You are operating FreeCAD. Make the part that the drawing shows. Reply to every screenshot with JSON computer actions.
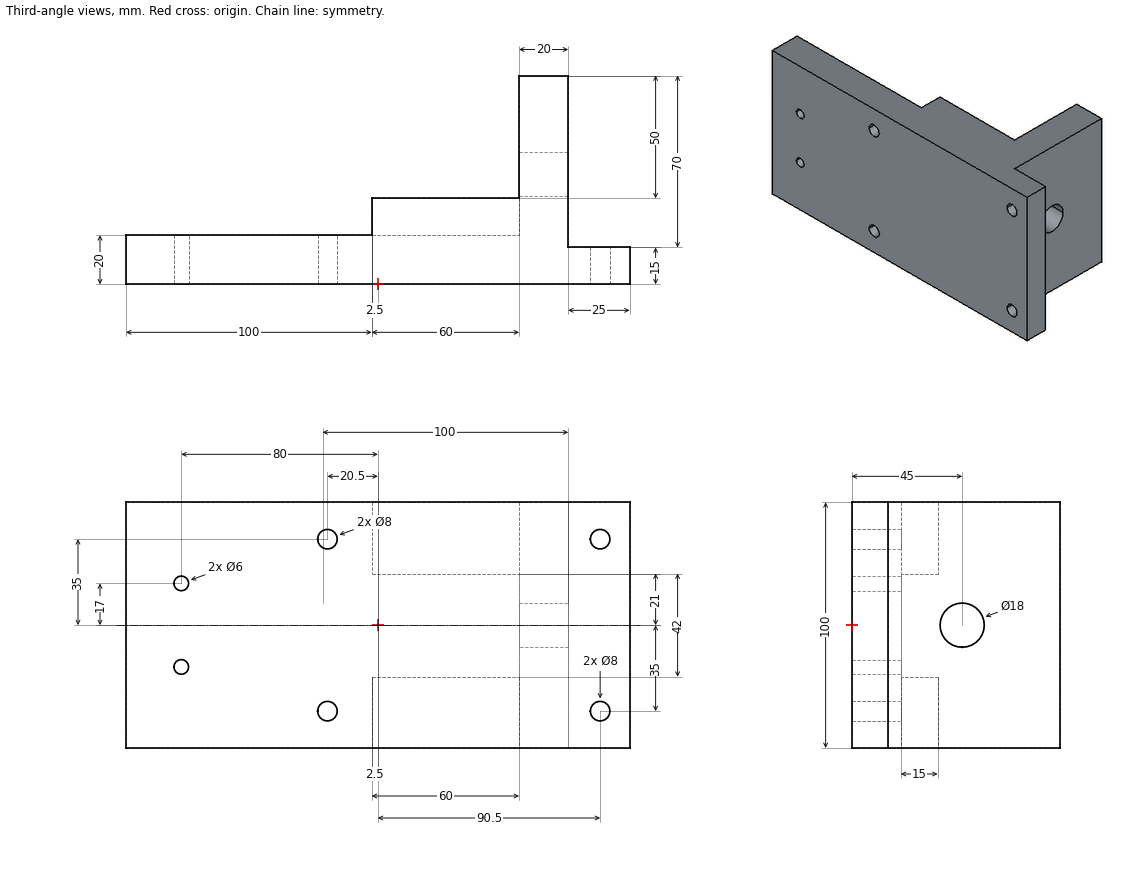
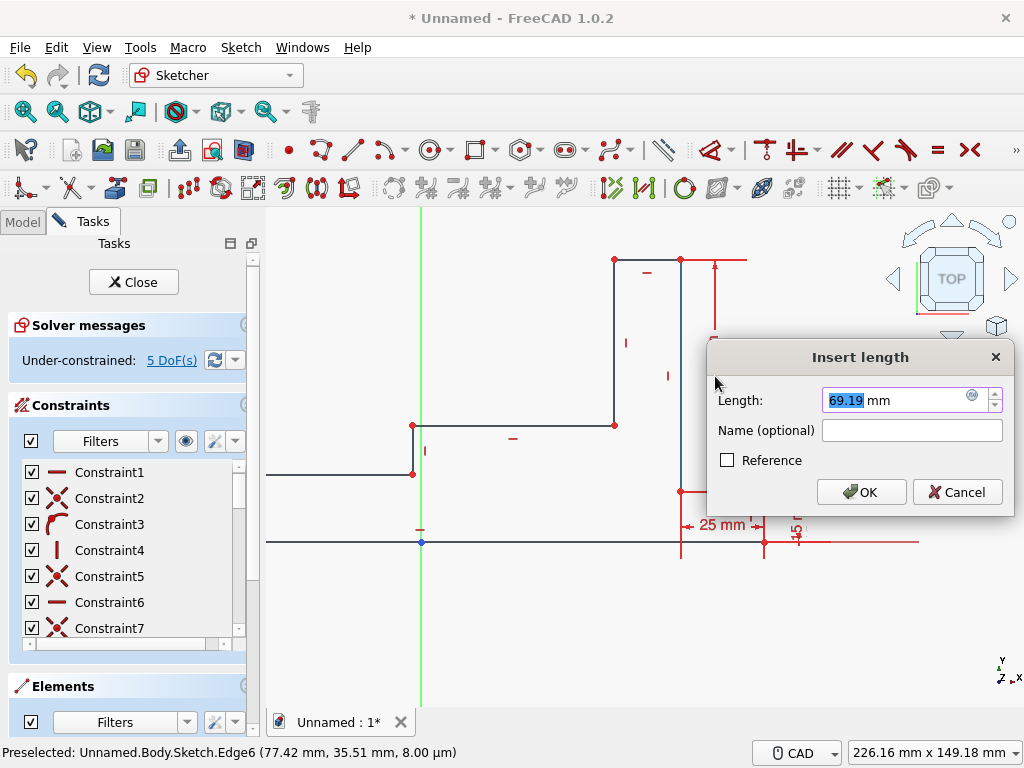
{"action": "type", "text": "70"}
{"action": "key", "text": "Return"}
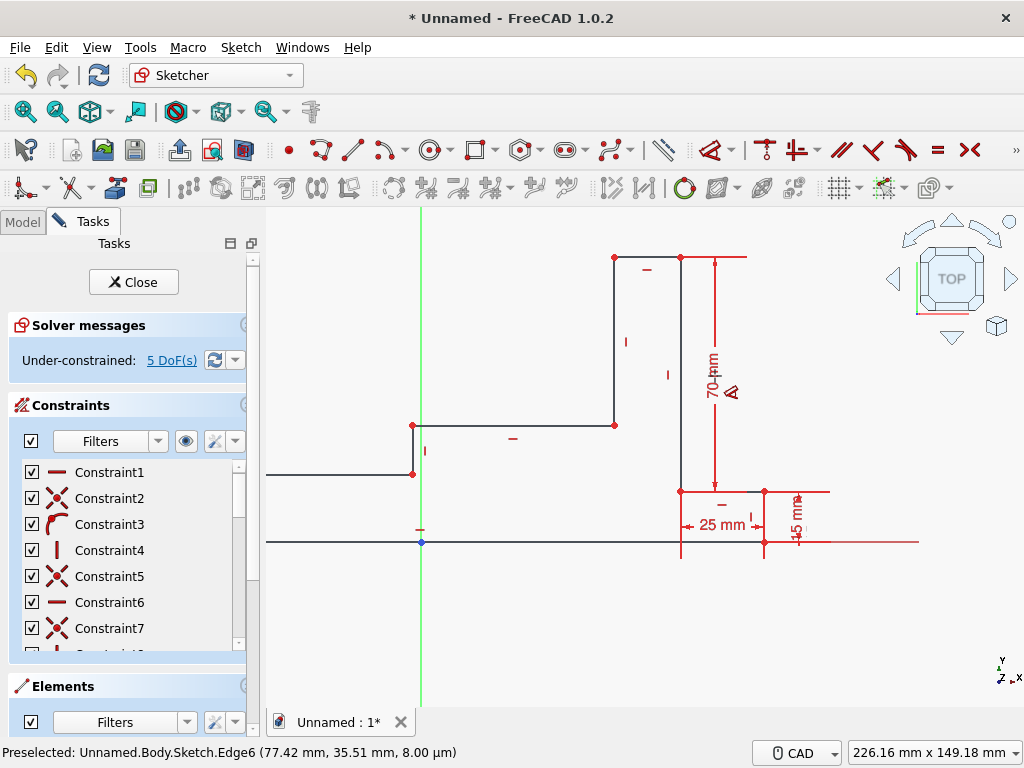
{"action": "left_click", "coordinate": [661, 257]}
{"action": "left_click", "coordinate": [648, 291]}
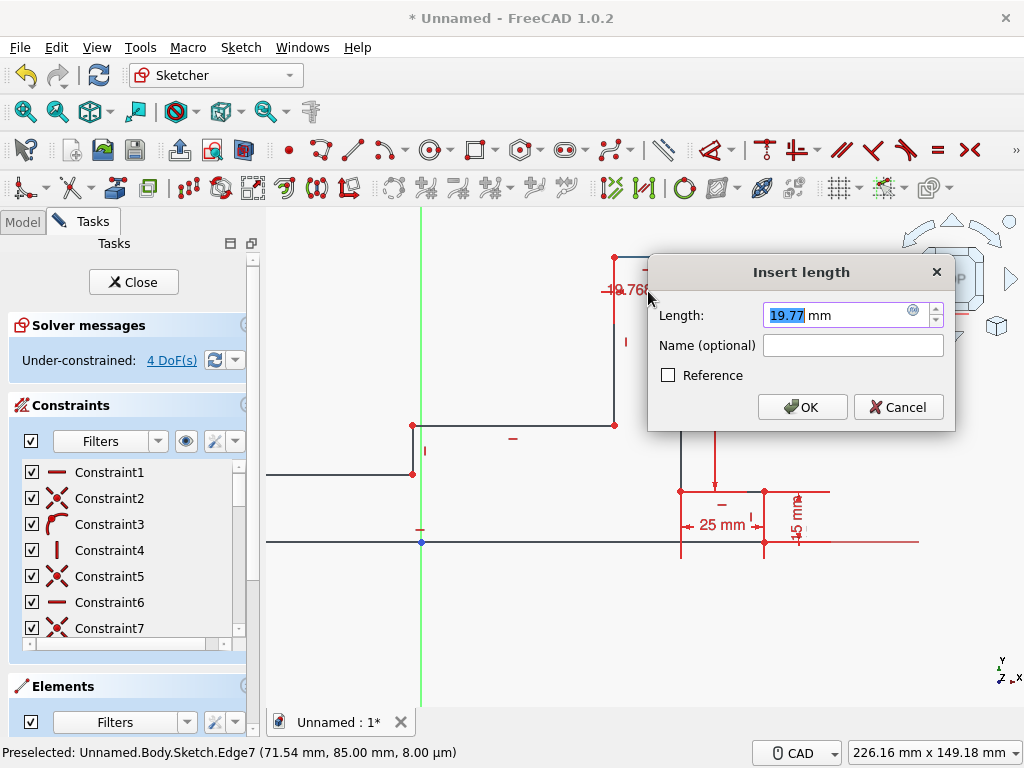
{"action": "type", "text": "20"}
{"action": "key", "text": "Return"}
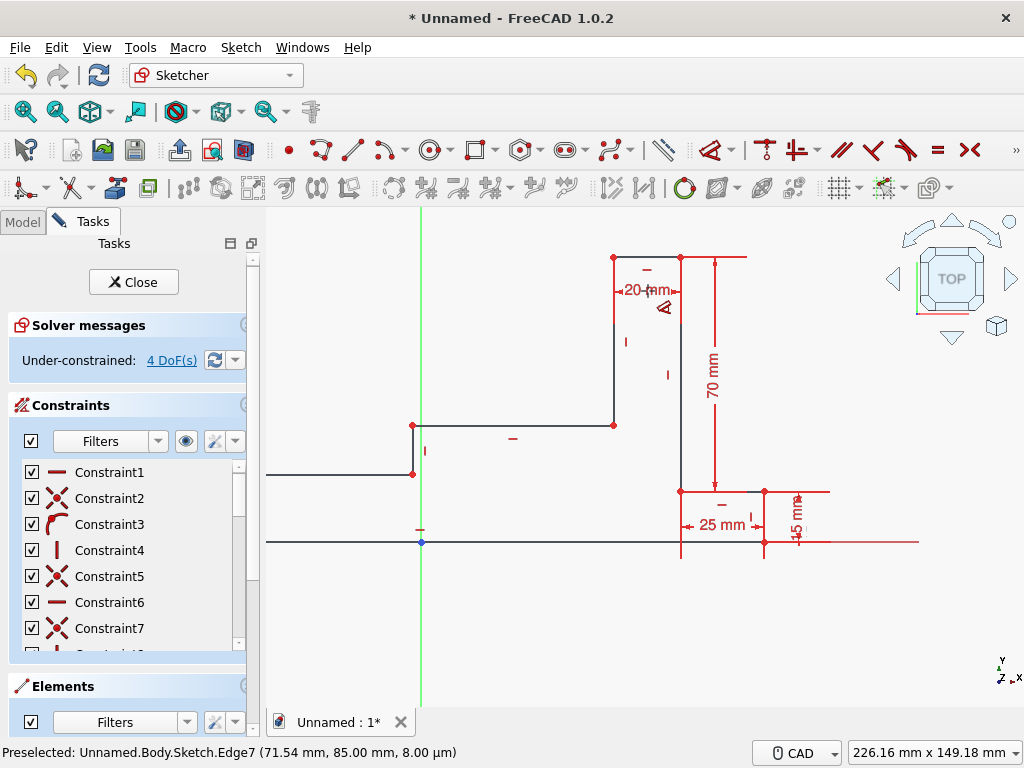
{"action": "left_click", "coordinate": [614, 308]}
{"action": "left_click", "coordinate": [648, 341]}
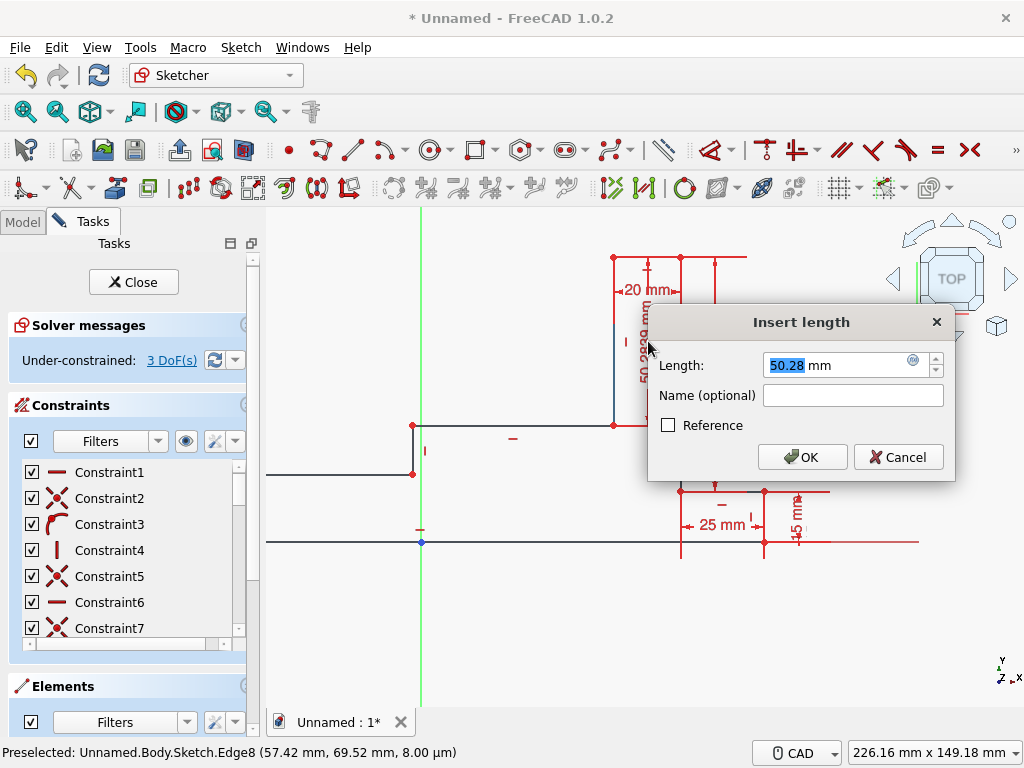
{"action": "type", "text": "50"}
{"action": "key", "text": "Return"}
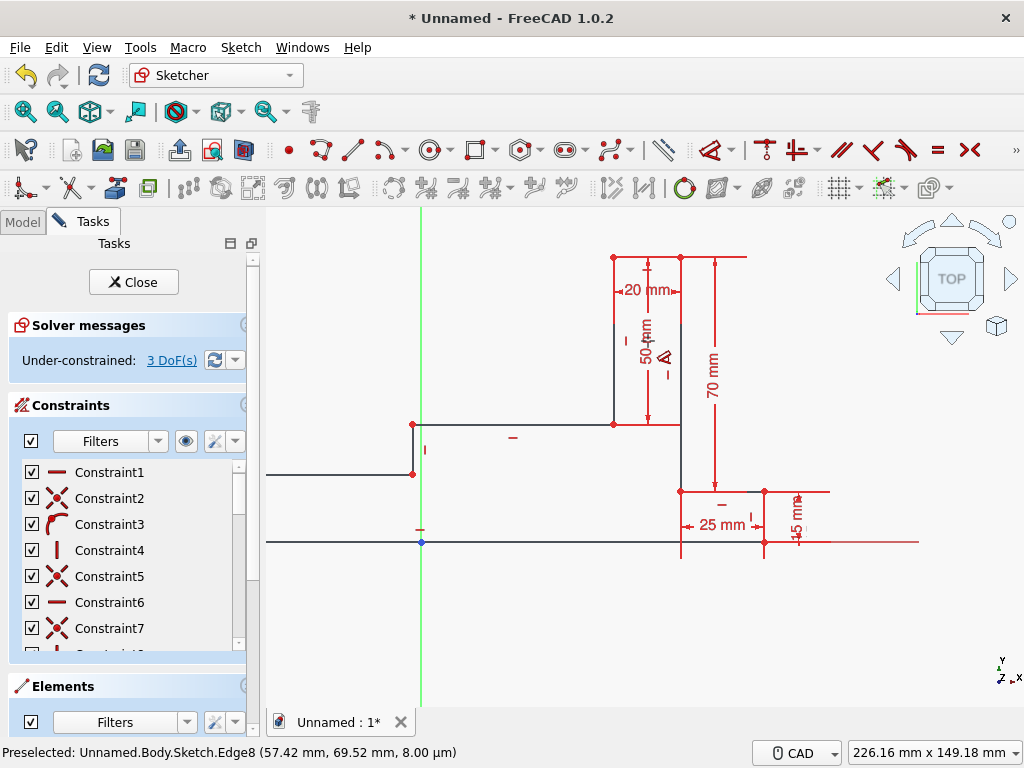
{"action": "left_click", "coordinate": [553, 425]}
{"action": "left_click", "coordinate": [513, 459]}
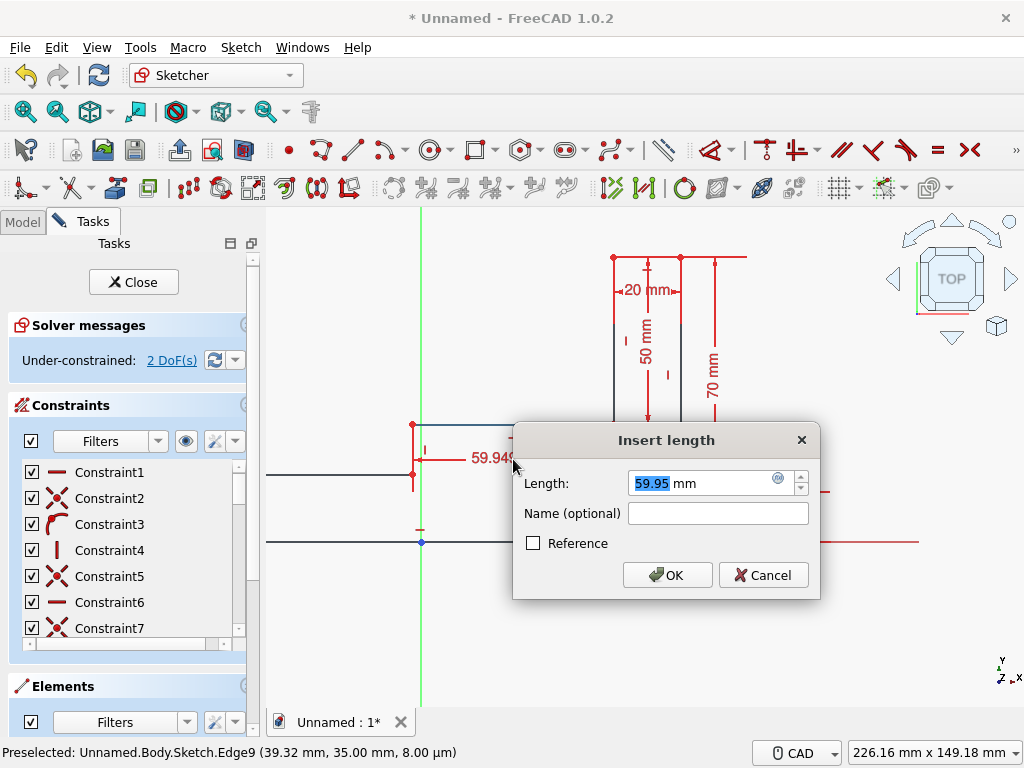
{"action": "type", "text": "60"}
{"action": "key", "text": "Return"}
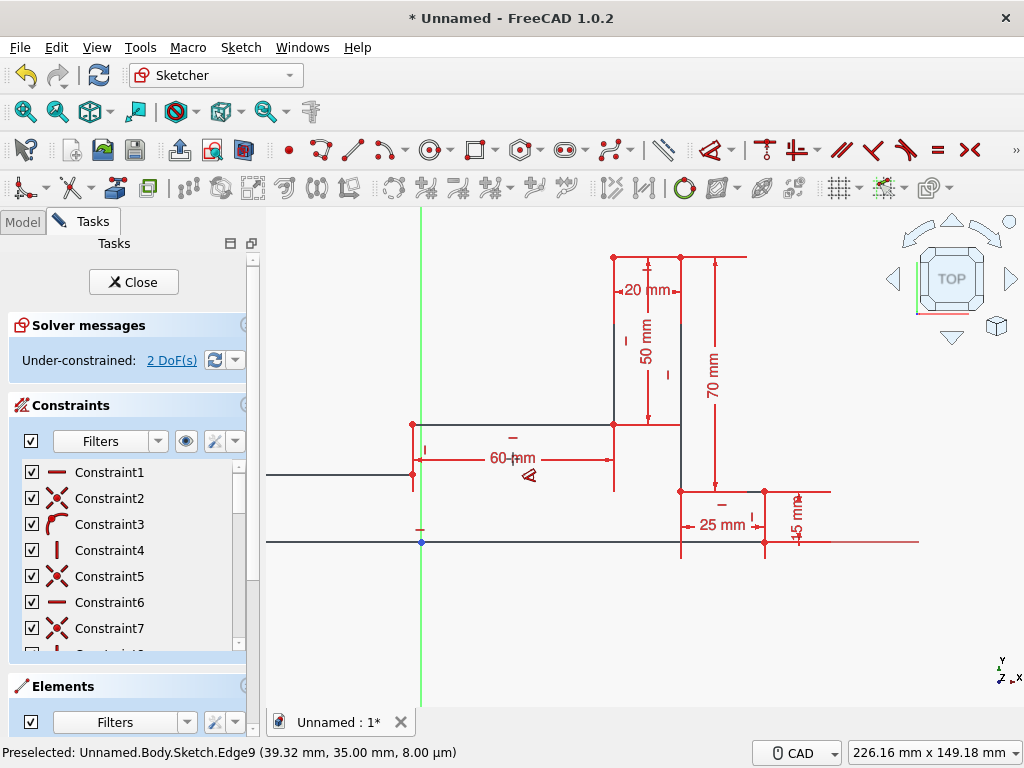
{"action": "left_click", "coordinate": [312, 475]}
{"action": "left_click", "coordinate": [353, 509]}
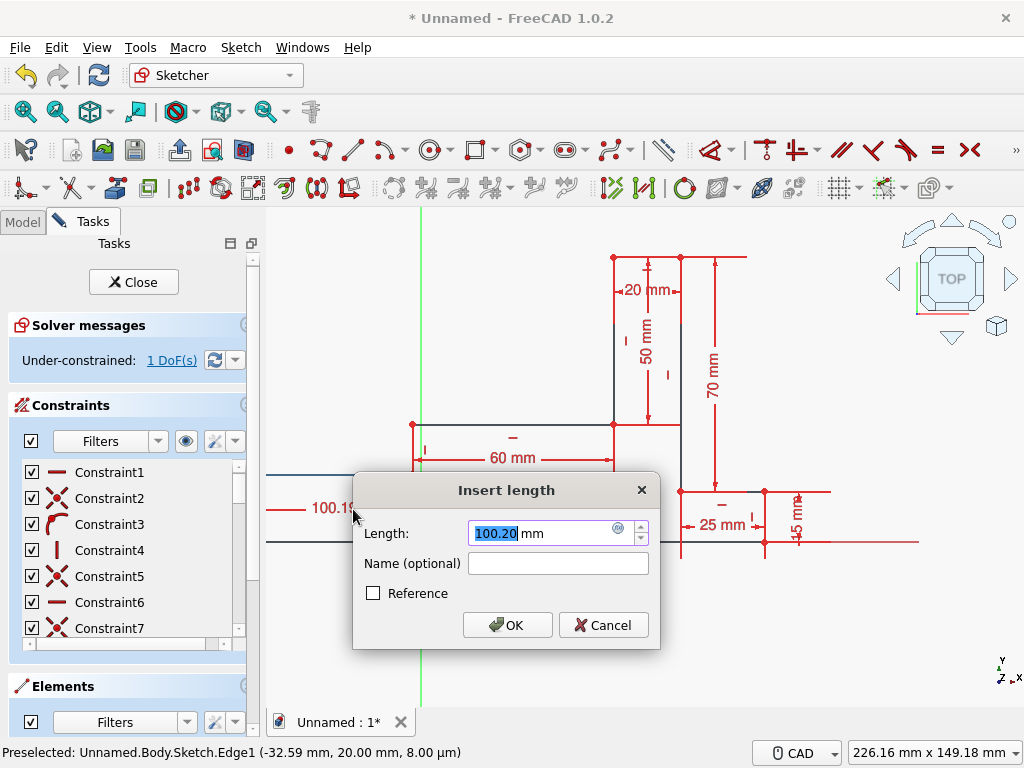
{"action": "type", "text": "100"}
{"action": "key", "text": "Return"}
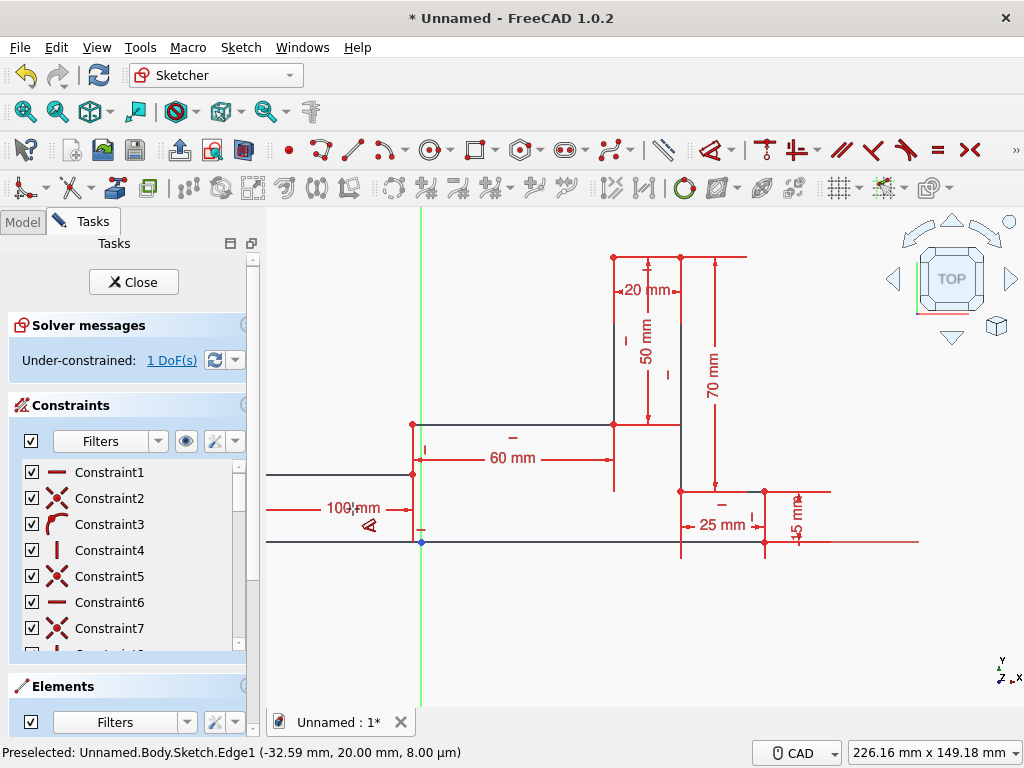
{"action": "scroll", "coordinate": [413, 475], "scroll_direction": "up", "scroll_amount": 8}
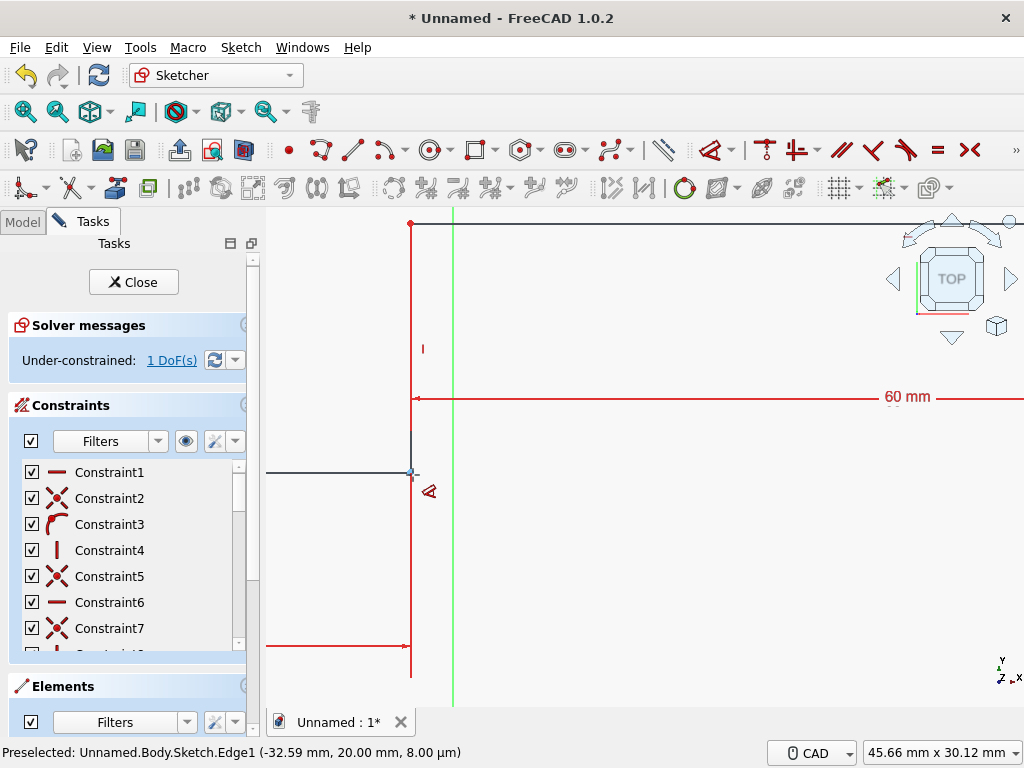
{"action": "left_click", "coordinate": [411, 473]}
{"action": "left_click", "coordinate": [432, 439]}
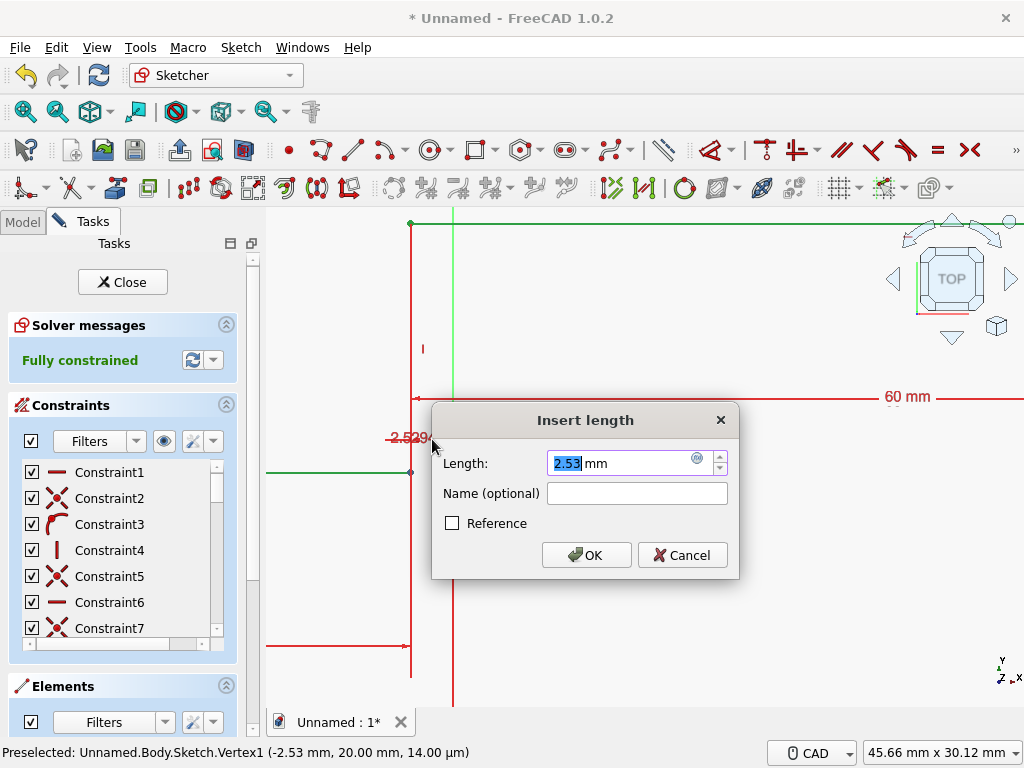
{"action": "type", "text": "2.5"}
{"action": "key", "text": "Return"}
{"action": "key", "text": "Escape"}